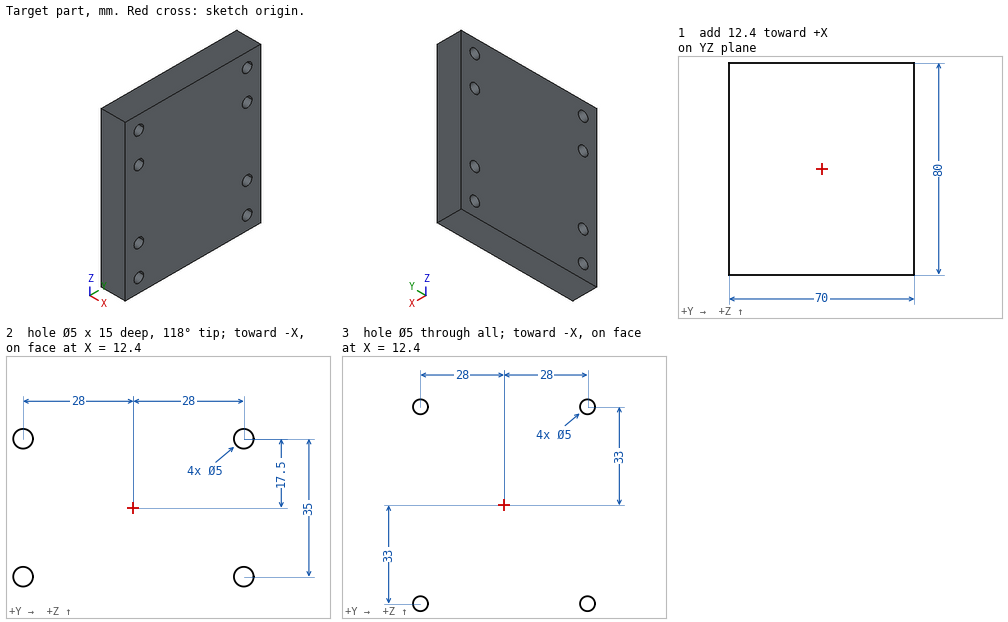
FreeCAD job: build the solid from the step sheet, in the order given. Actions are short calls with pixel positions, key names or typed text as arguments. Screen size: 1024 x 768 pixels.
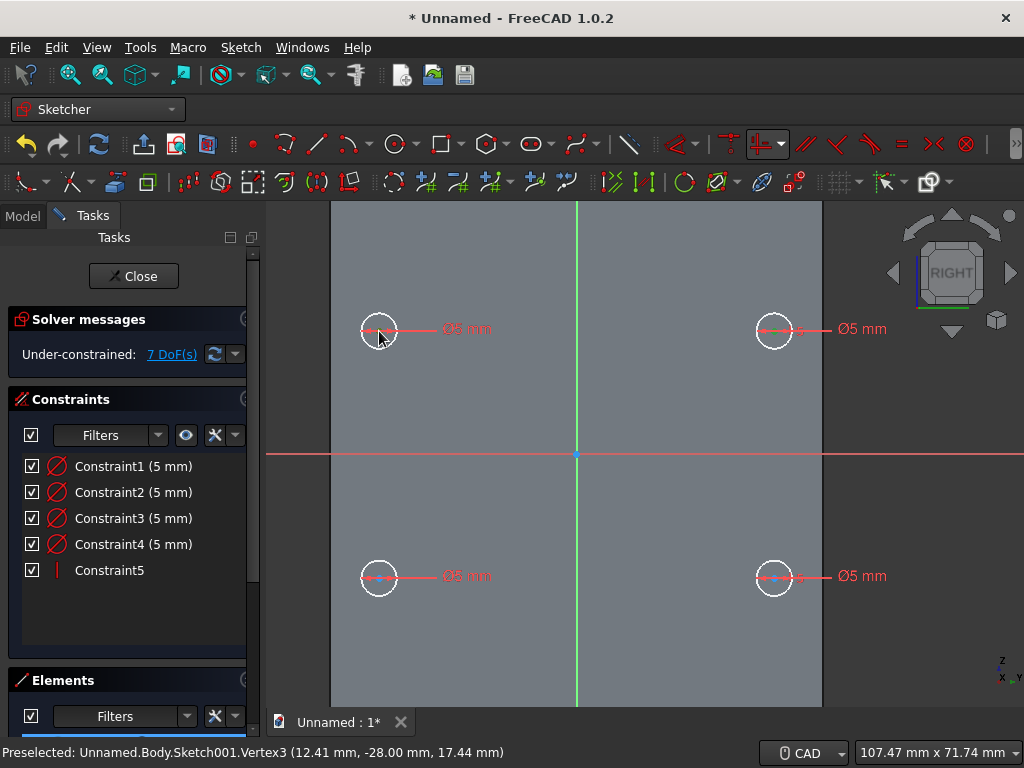
key(h)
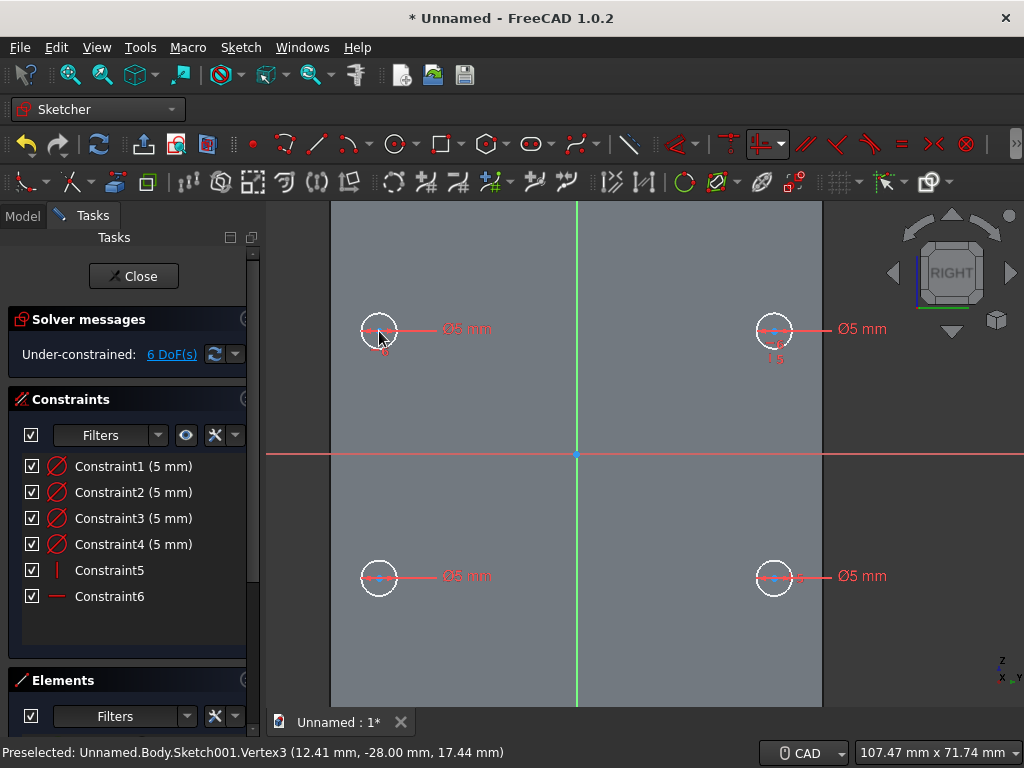
click(379, 331)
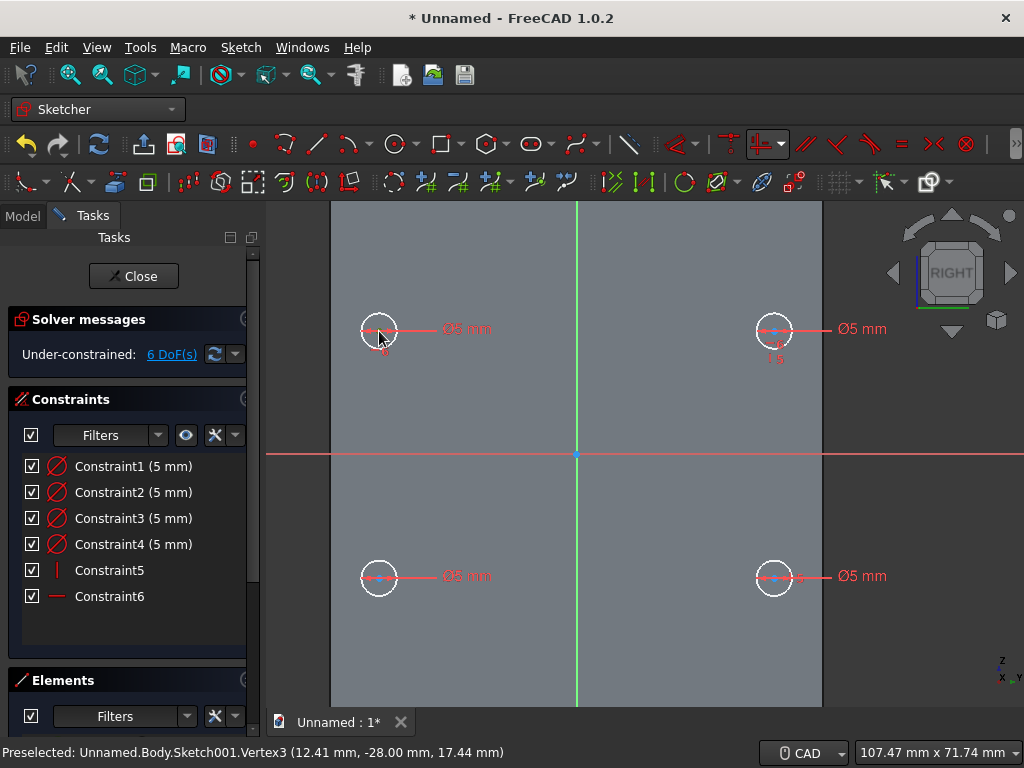
click(379, 578)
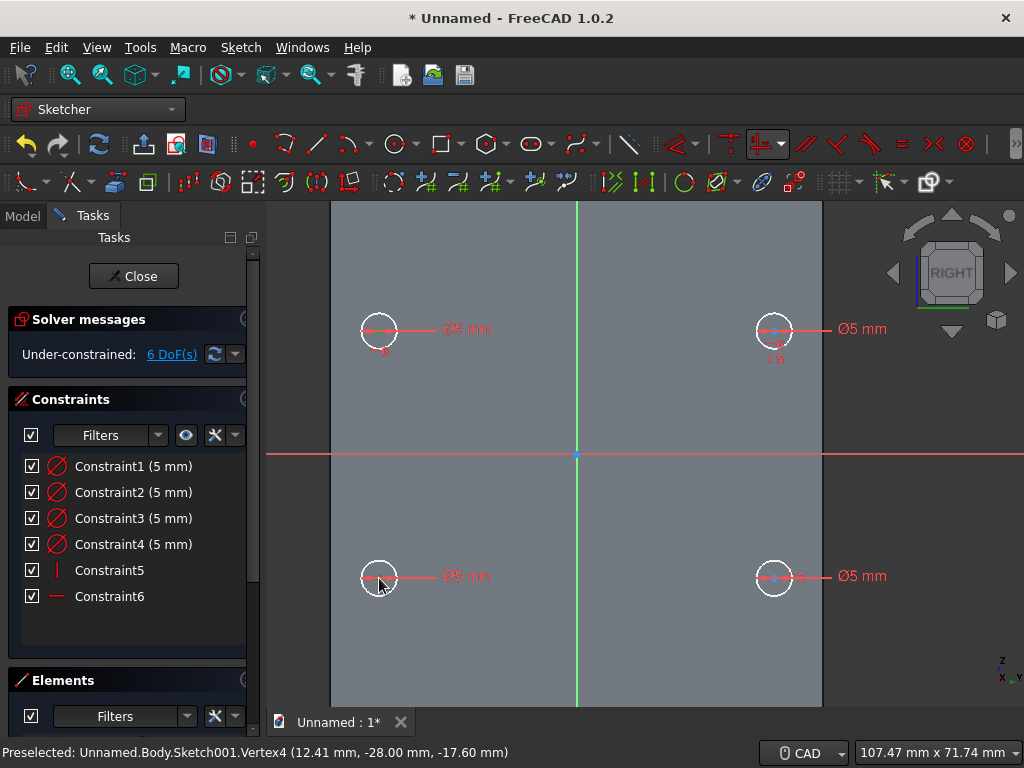
key(v)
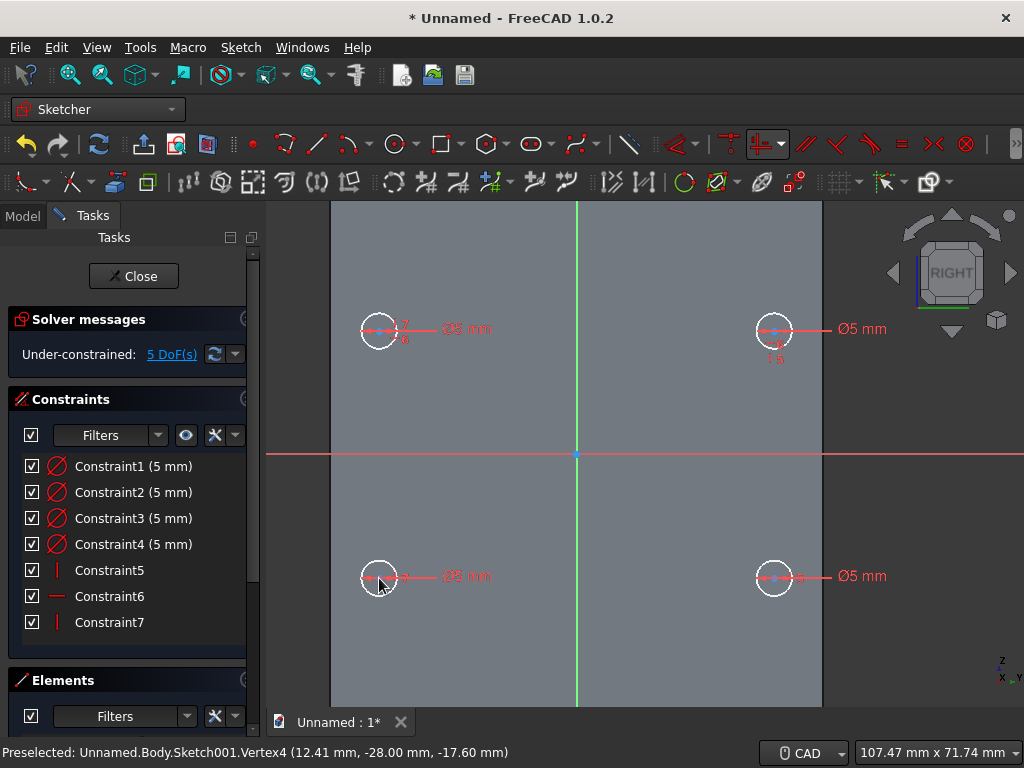
click(774, 578)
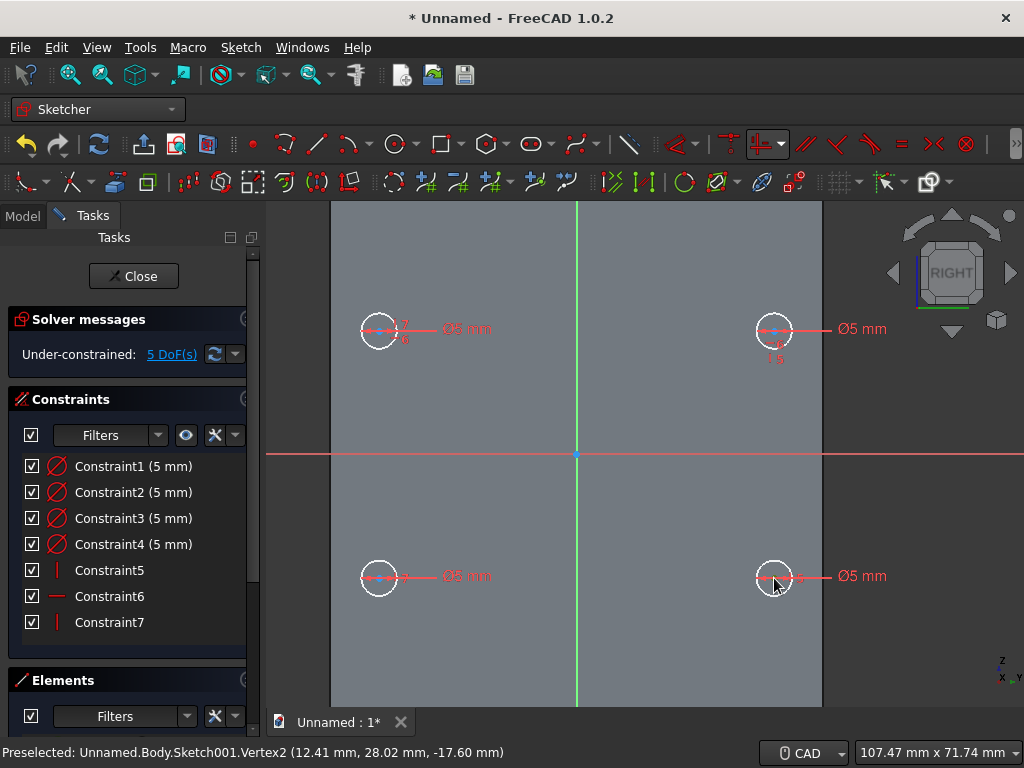
click(379, 578)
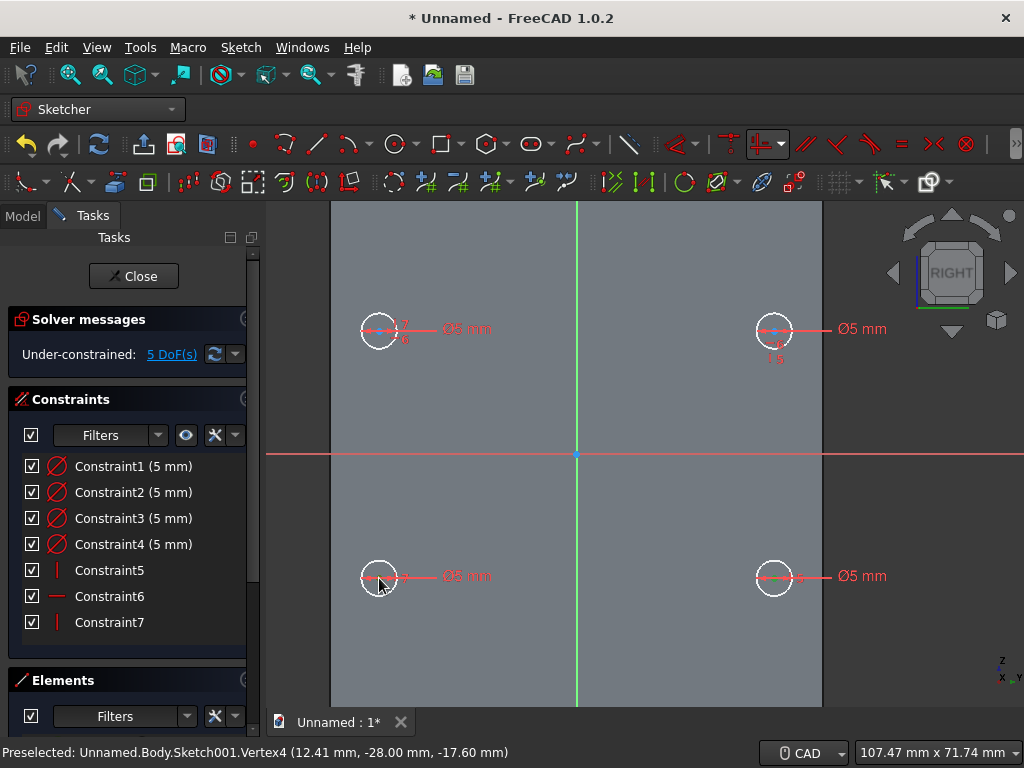
click(784, 144)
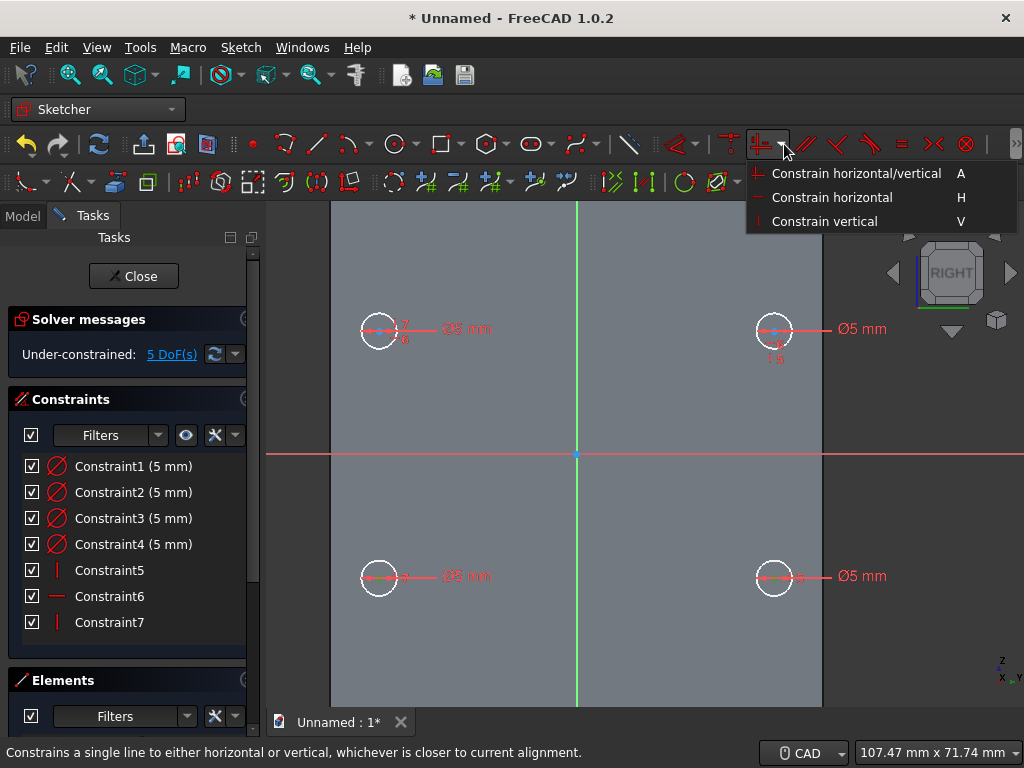
click(882, 197)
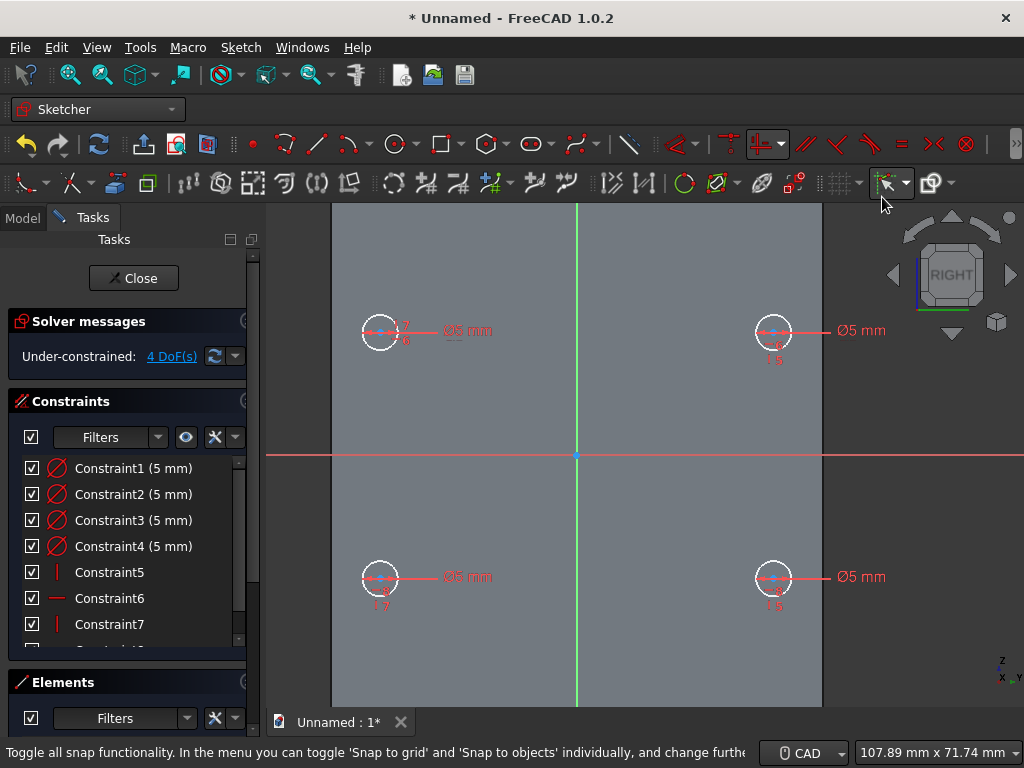
click(774, 333)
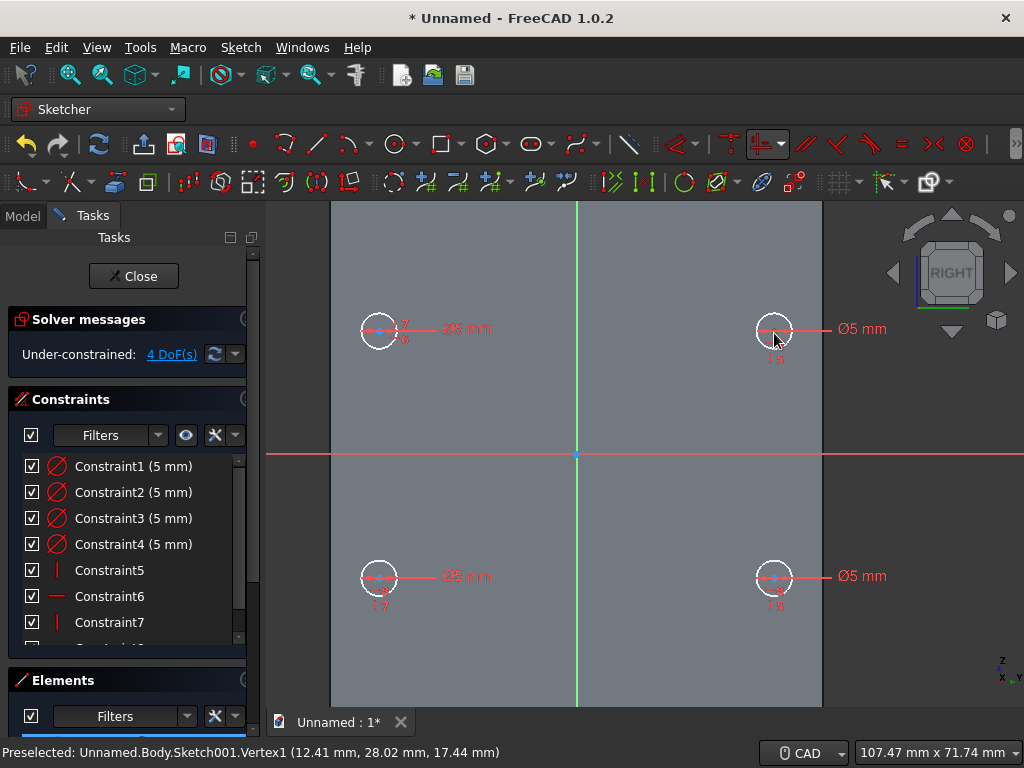
key(l)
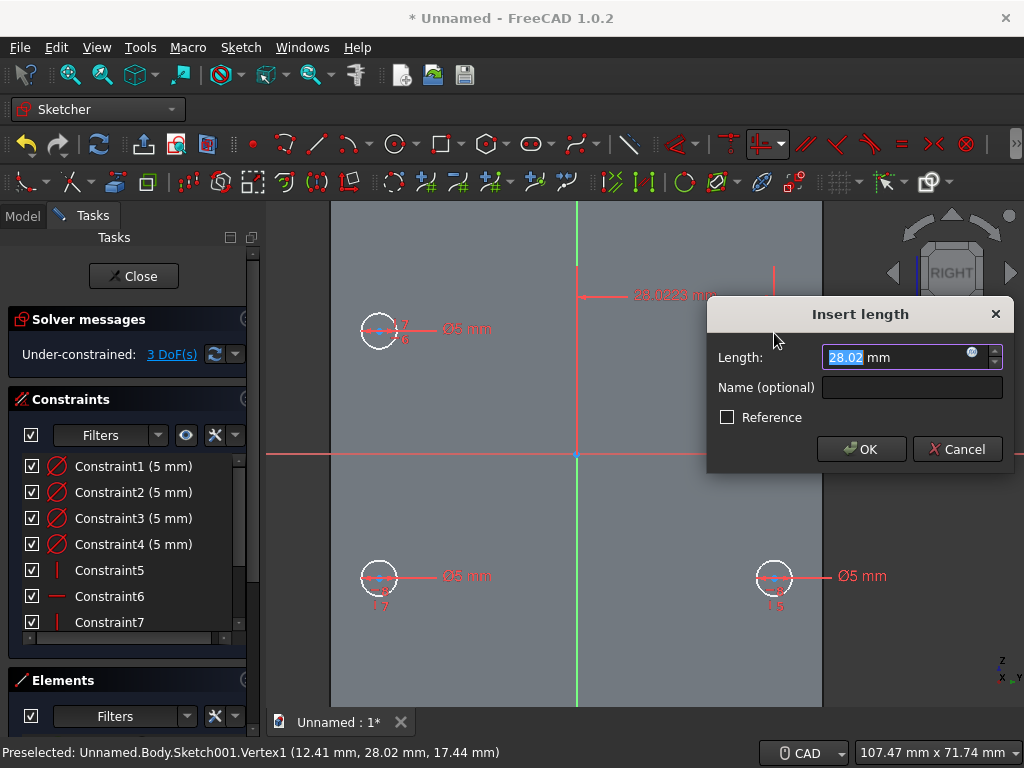
text(28)
key(Return)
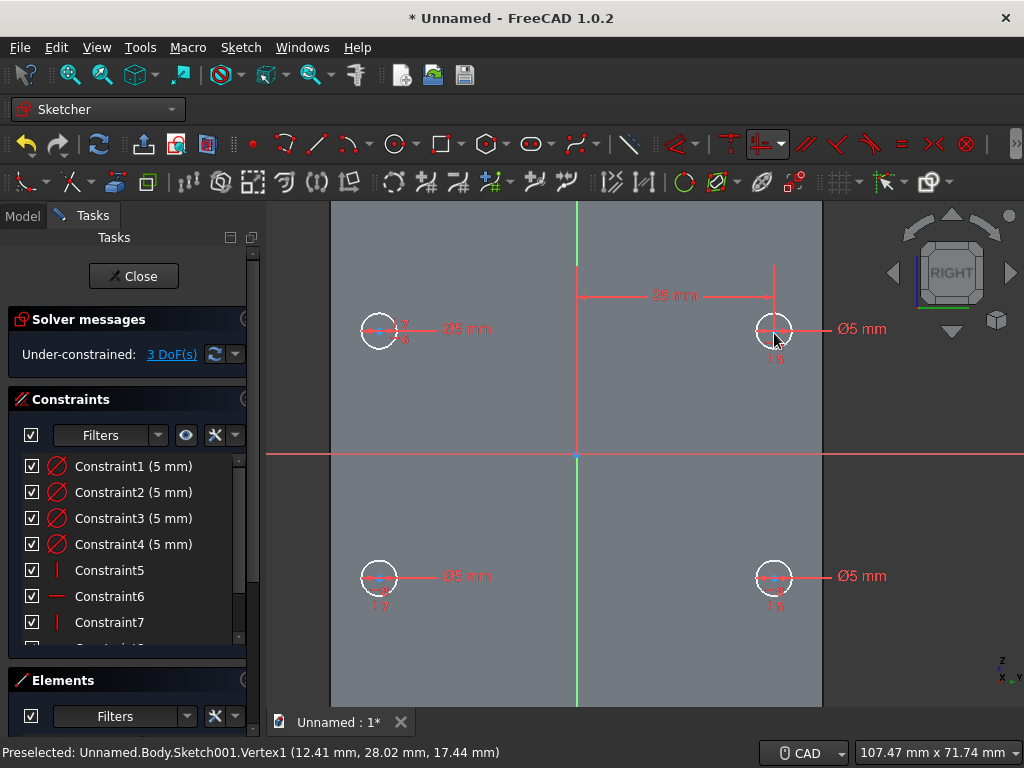
click(379, 331)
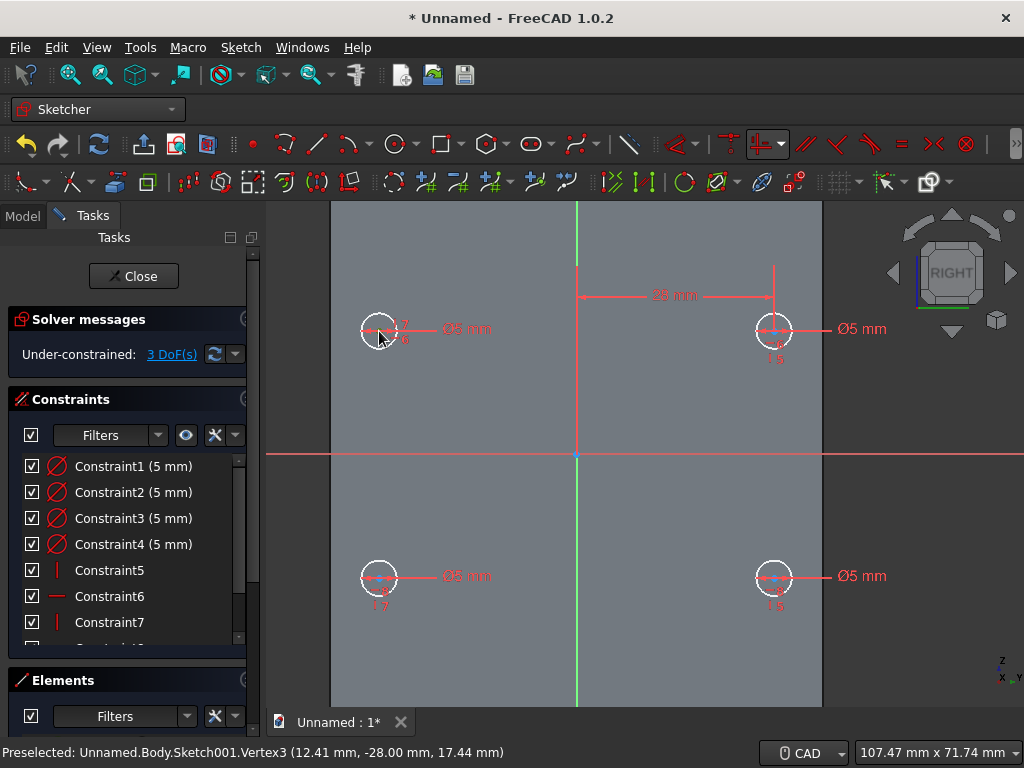
key(l)